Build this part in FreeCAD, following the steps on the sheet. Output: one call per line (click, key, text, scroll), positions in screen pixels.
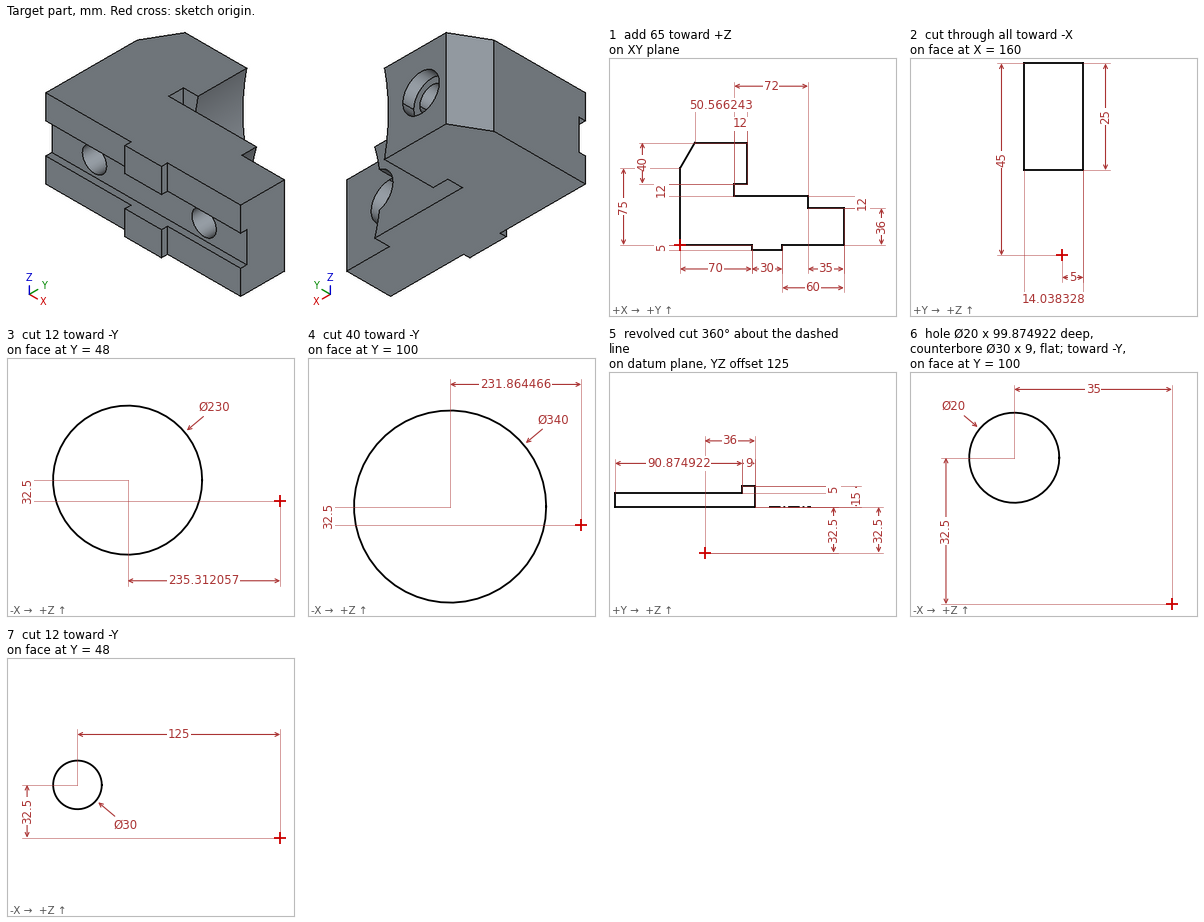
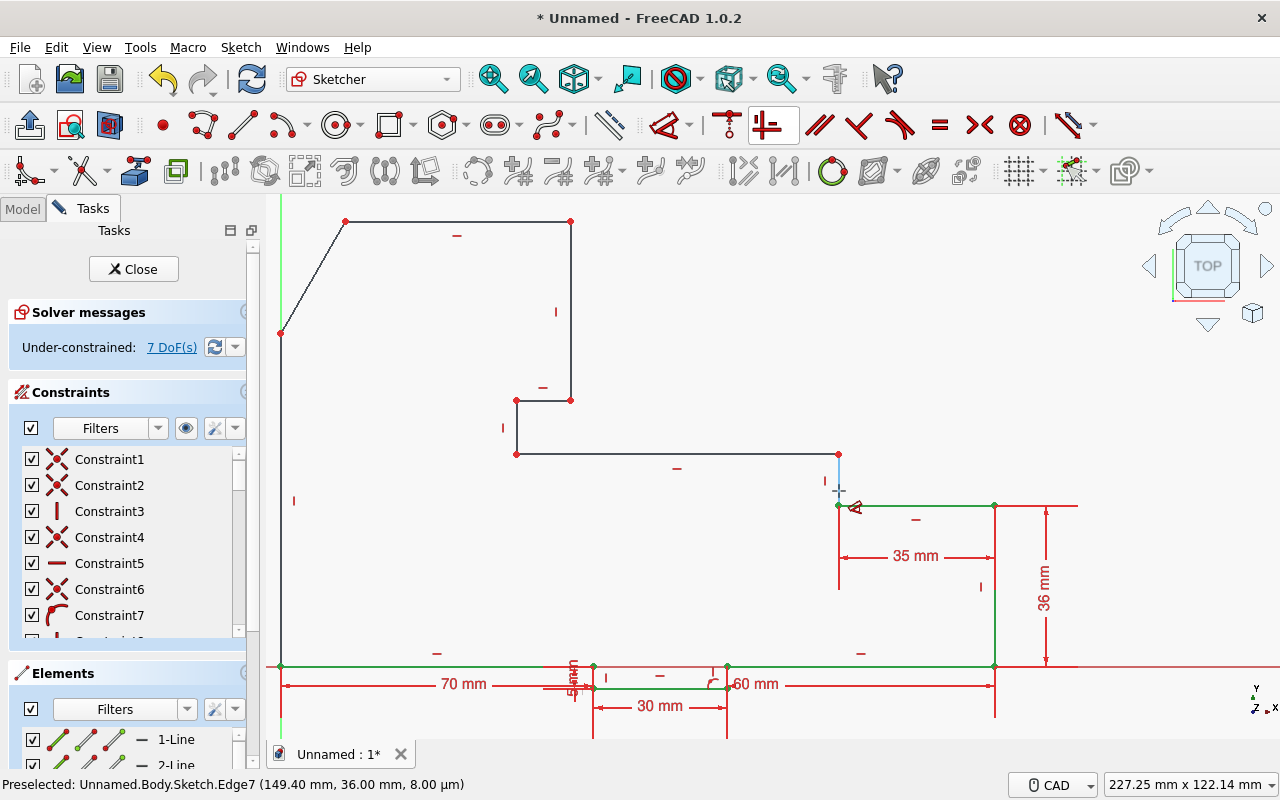
click(839, 491)
click(873, 480)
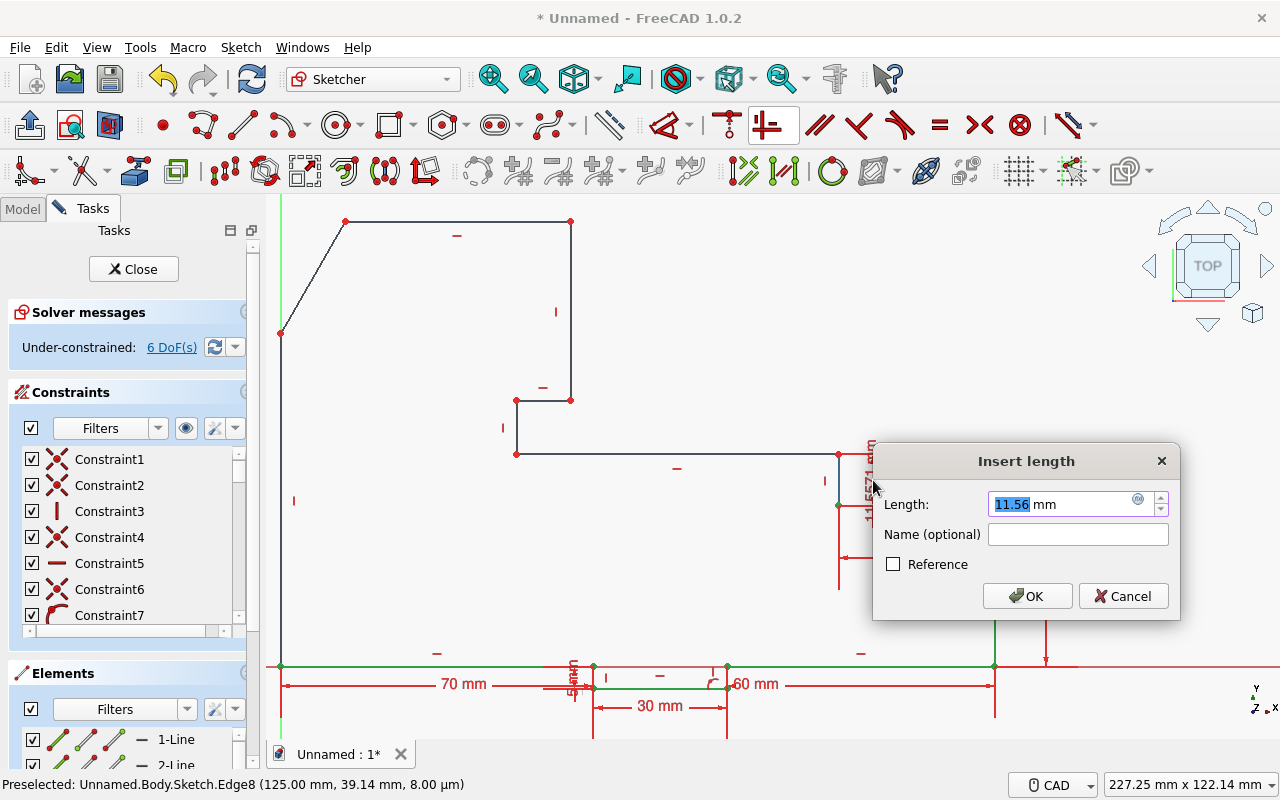
text(12)
key(Return)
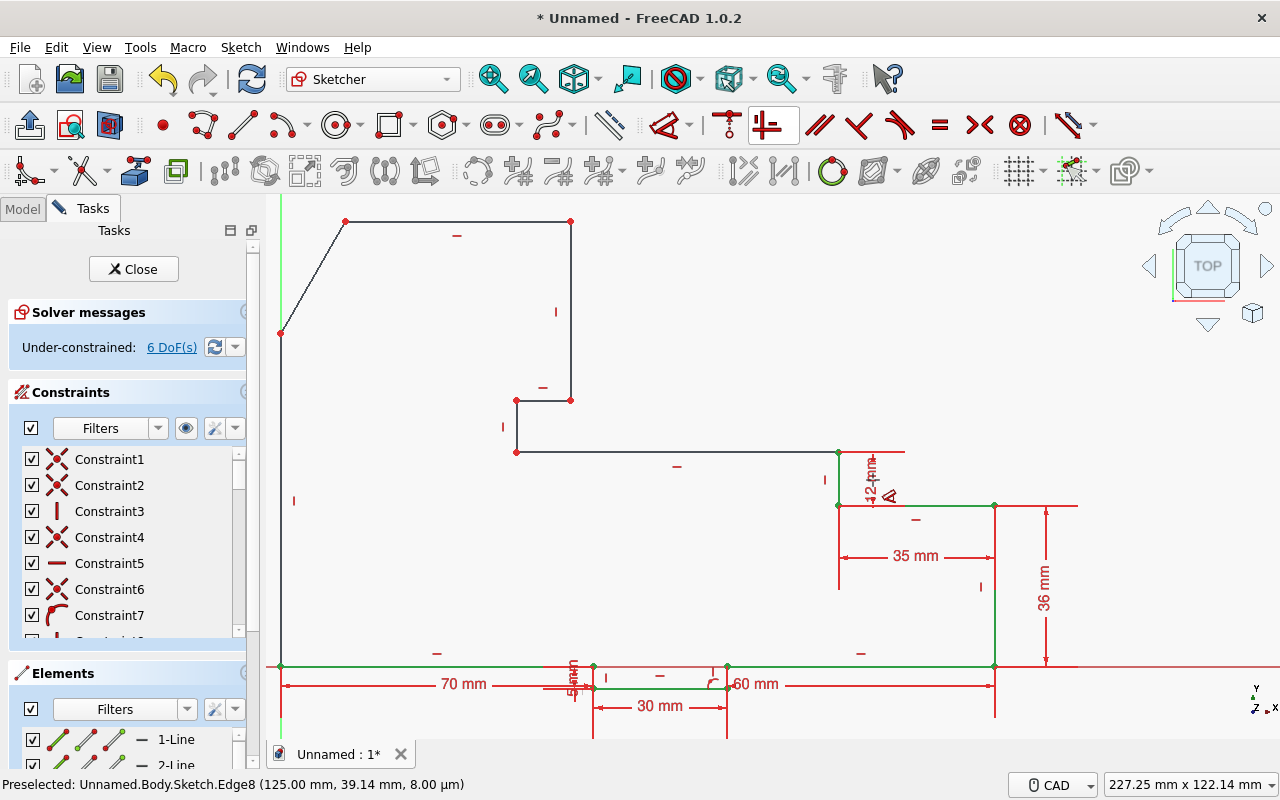
click(742, 452)
click(678, 418)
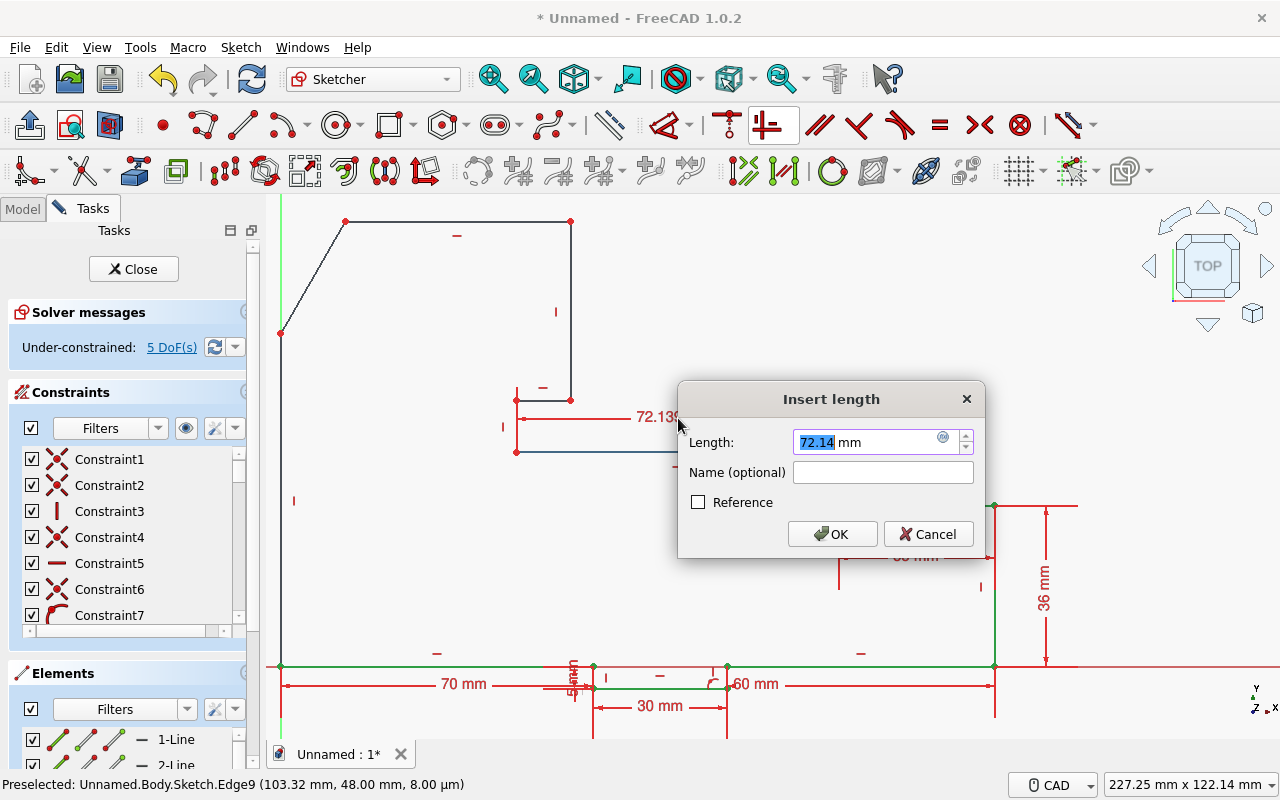
text(72)
key(Return)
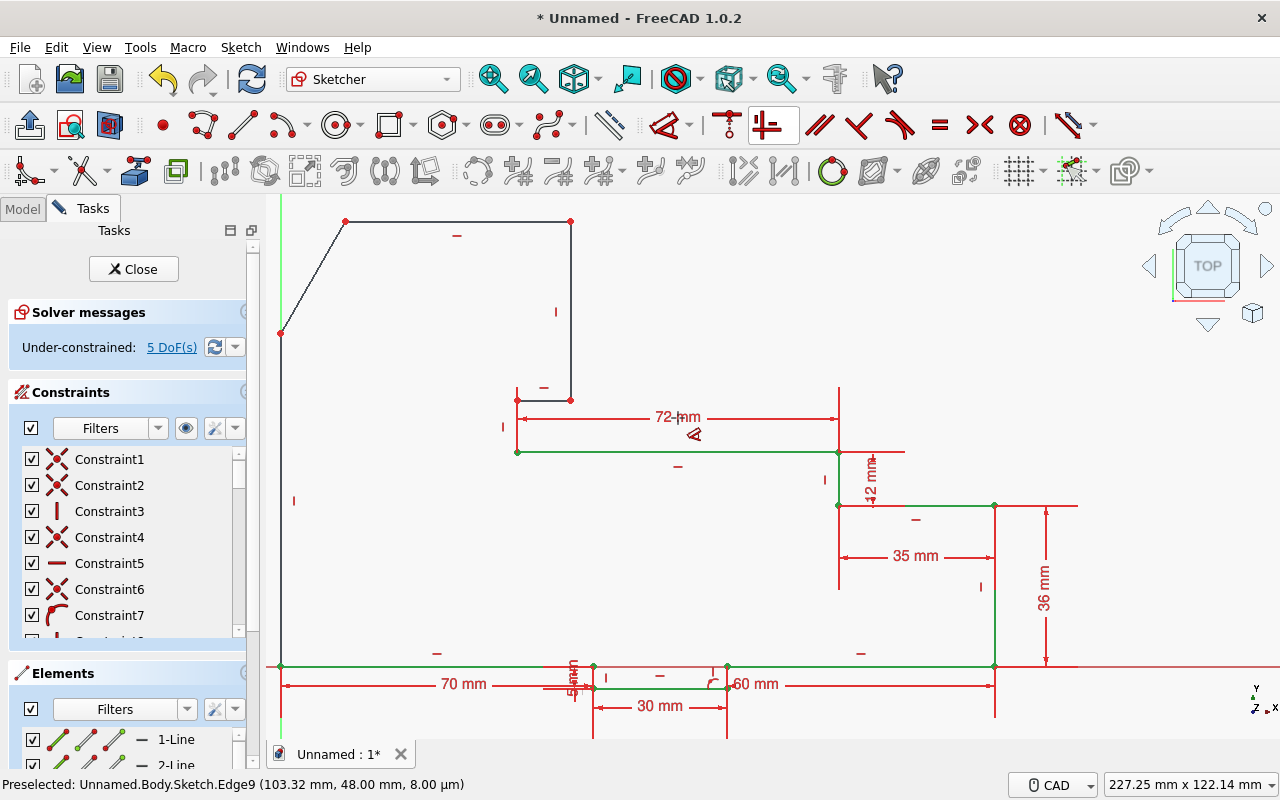
click(517, 437)
click(483, 427)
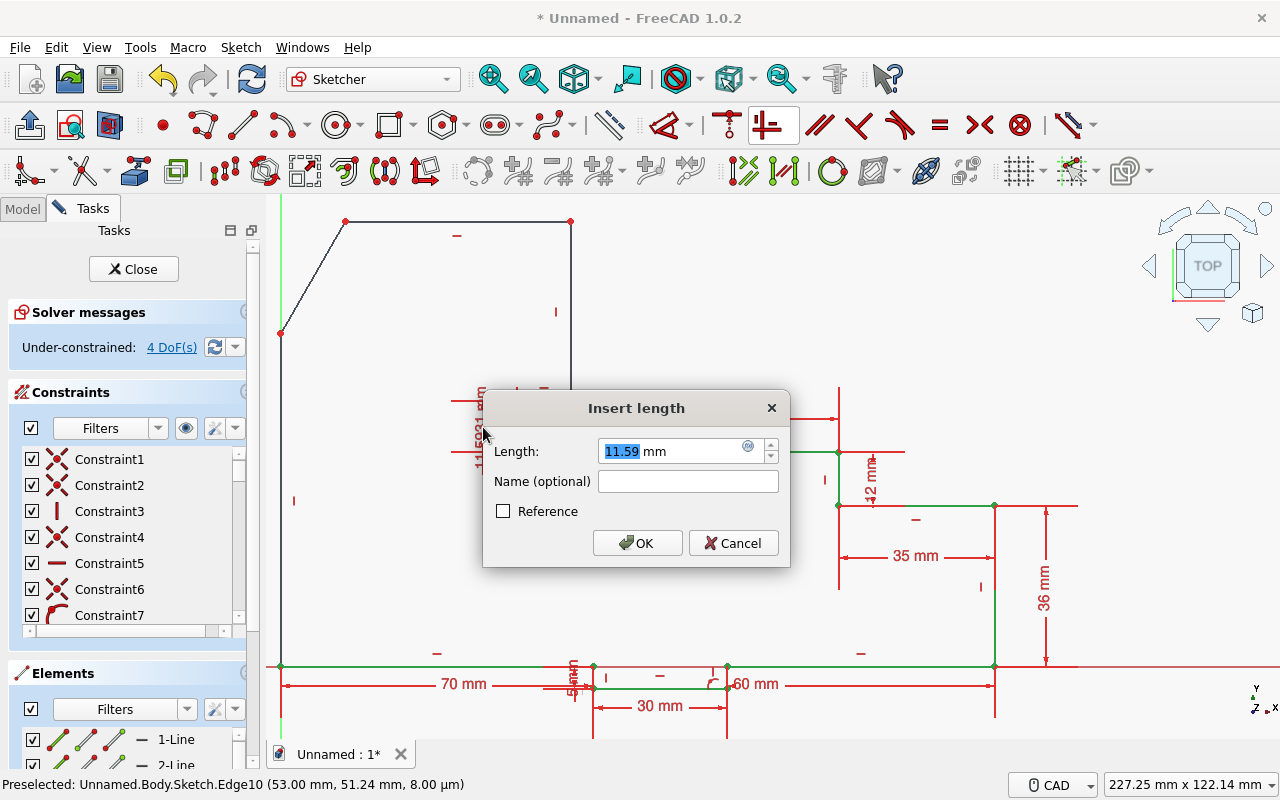
text(12)
key(Return)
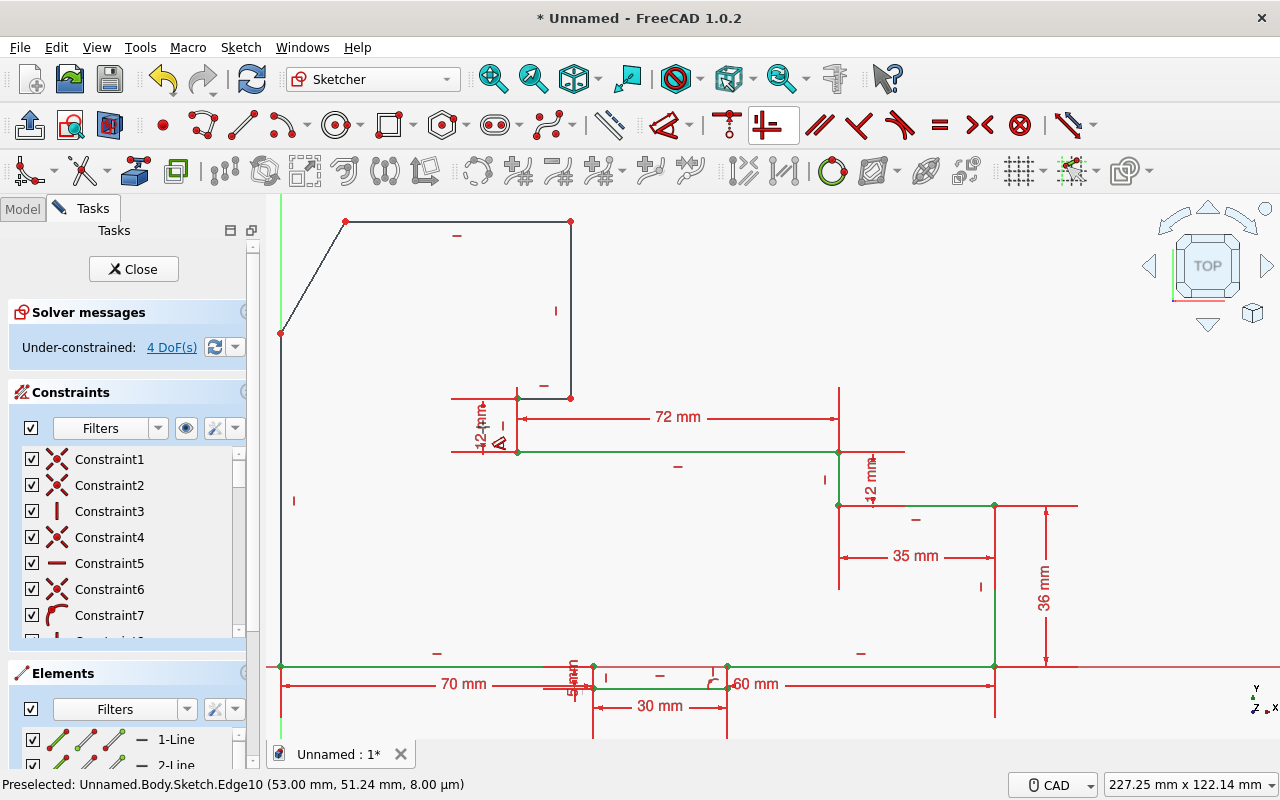
click(533, 399)
click(544, 365)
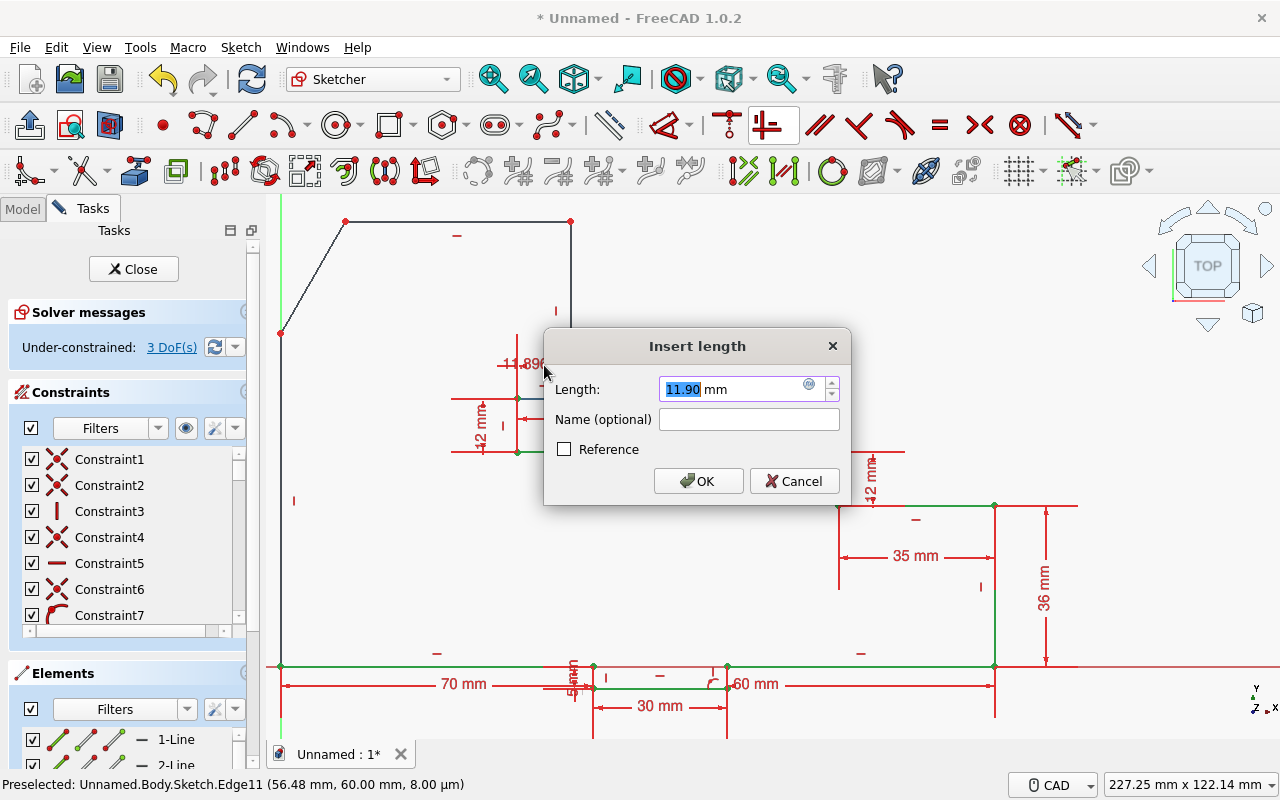
text(12)
key(Return)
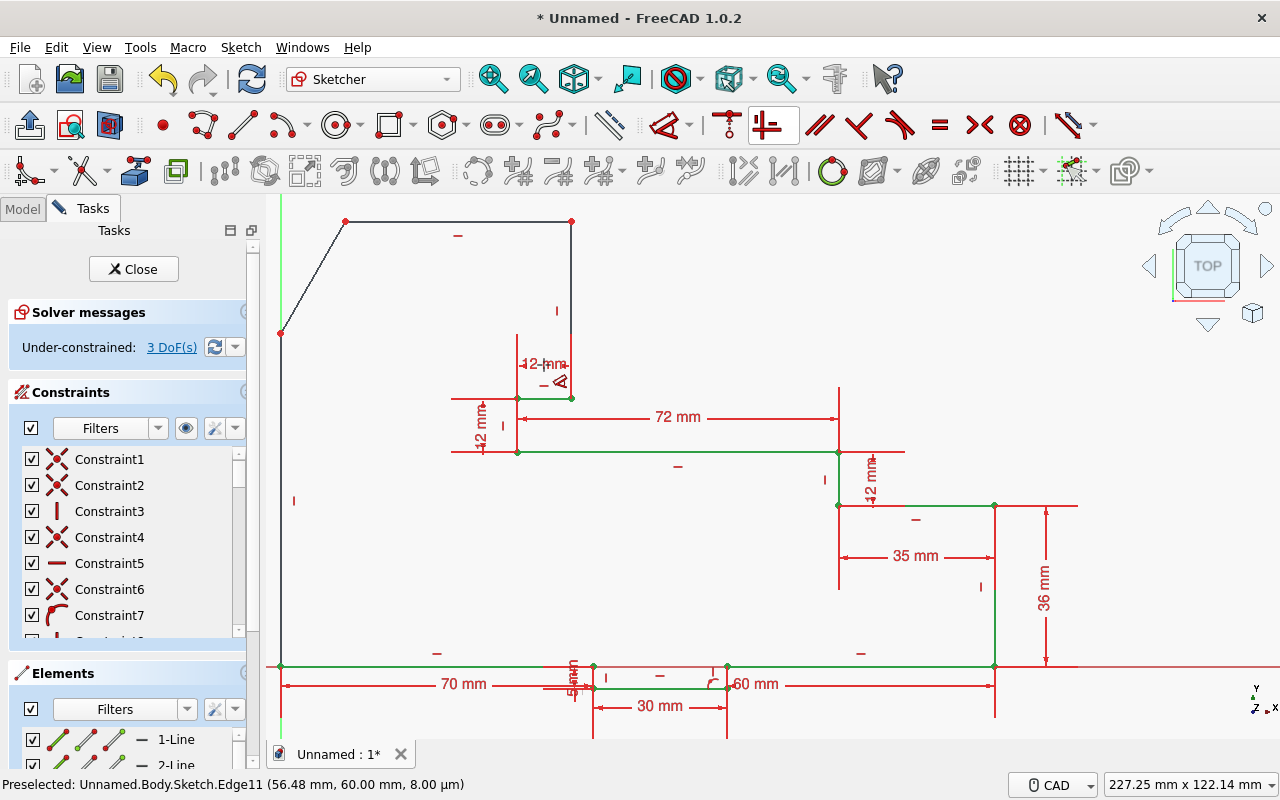
click(571, 346)
click(537, 310)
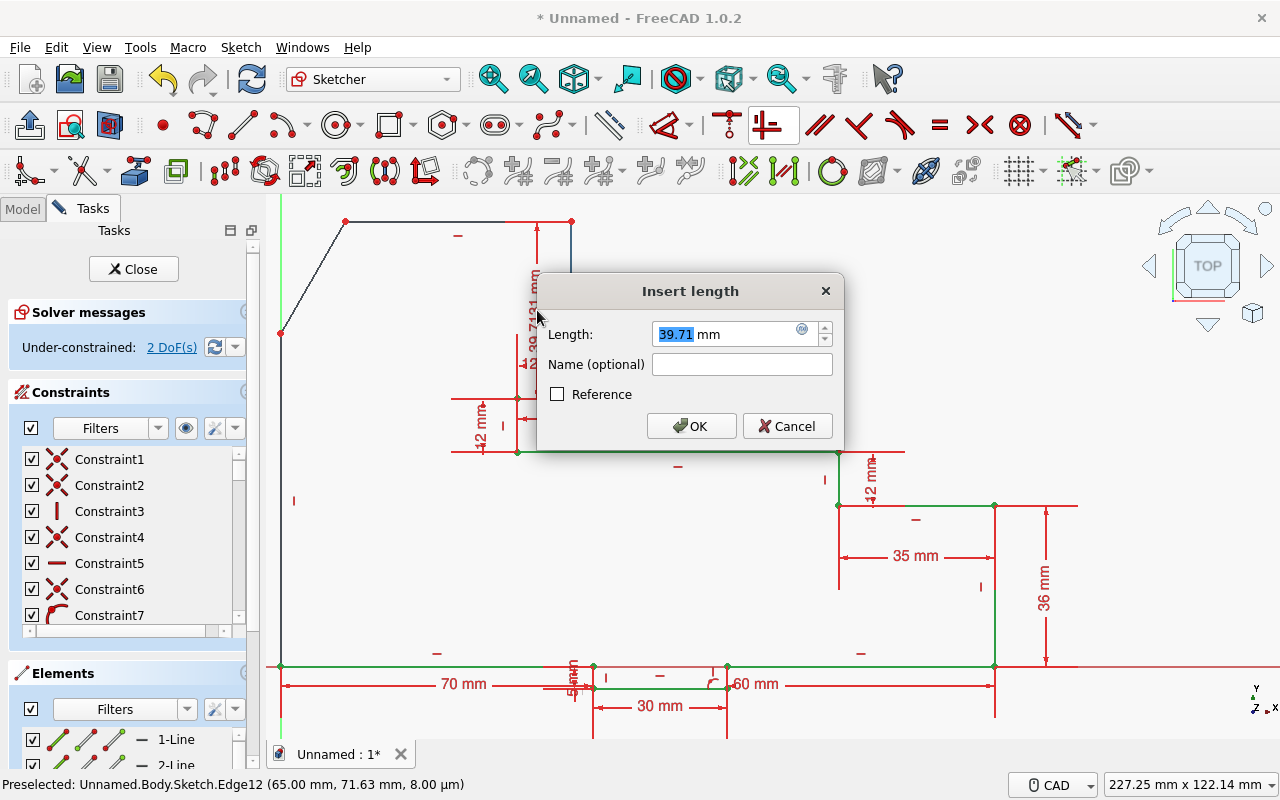
text(40)
key(Return)